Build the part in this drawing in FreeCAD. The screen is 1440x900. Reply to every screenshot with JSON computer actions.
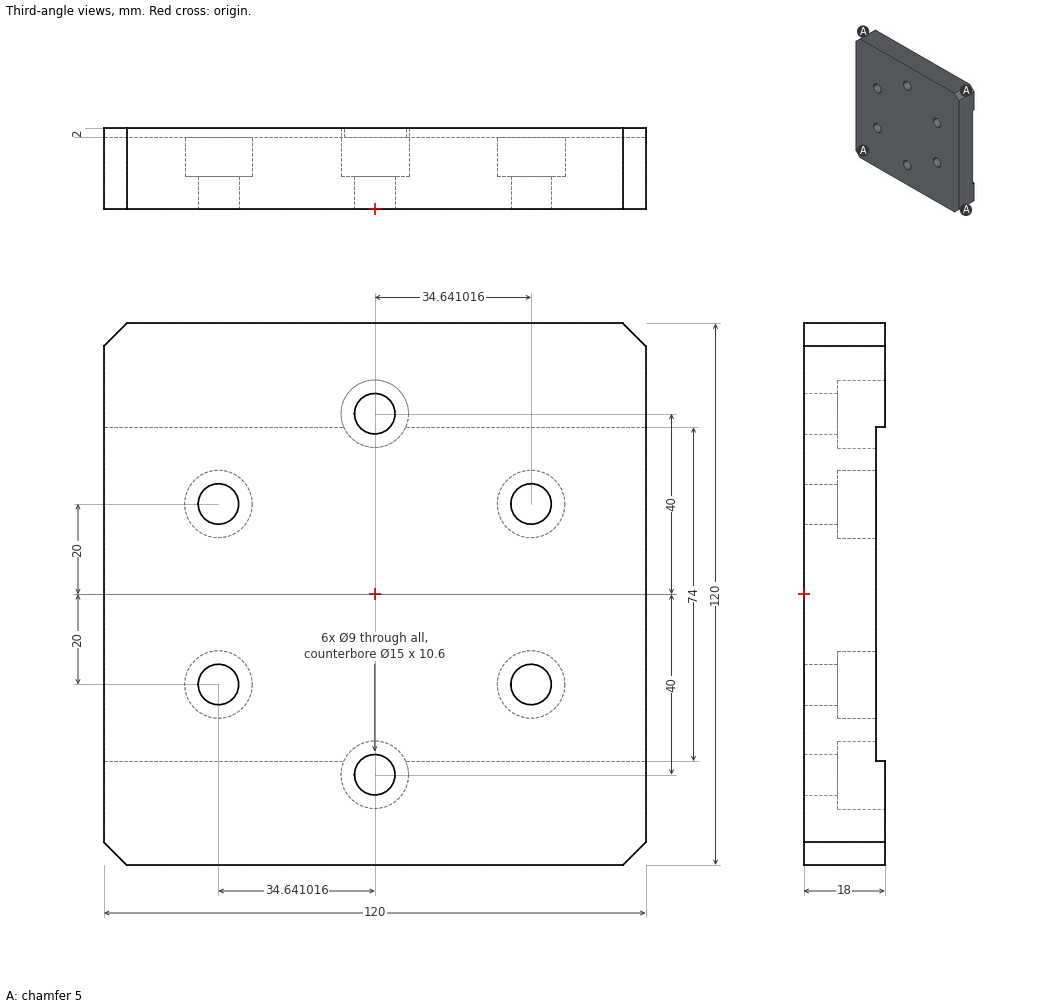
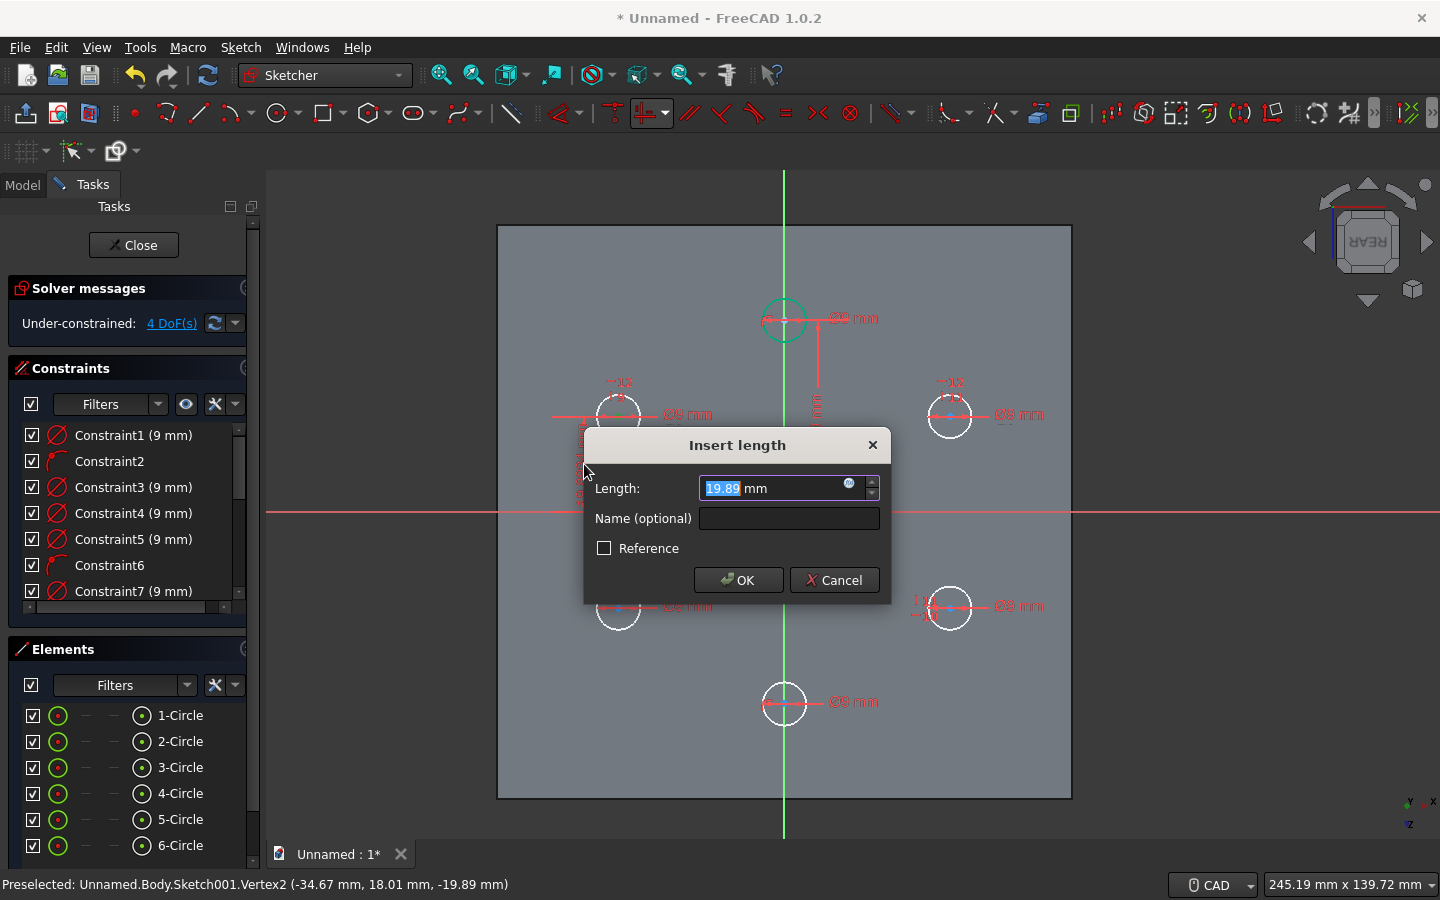
{"action": "type", "text": "20"}
{"action": "key", "text": "Return"}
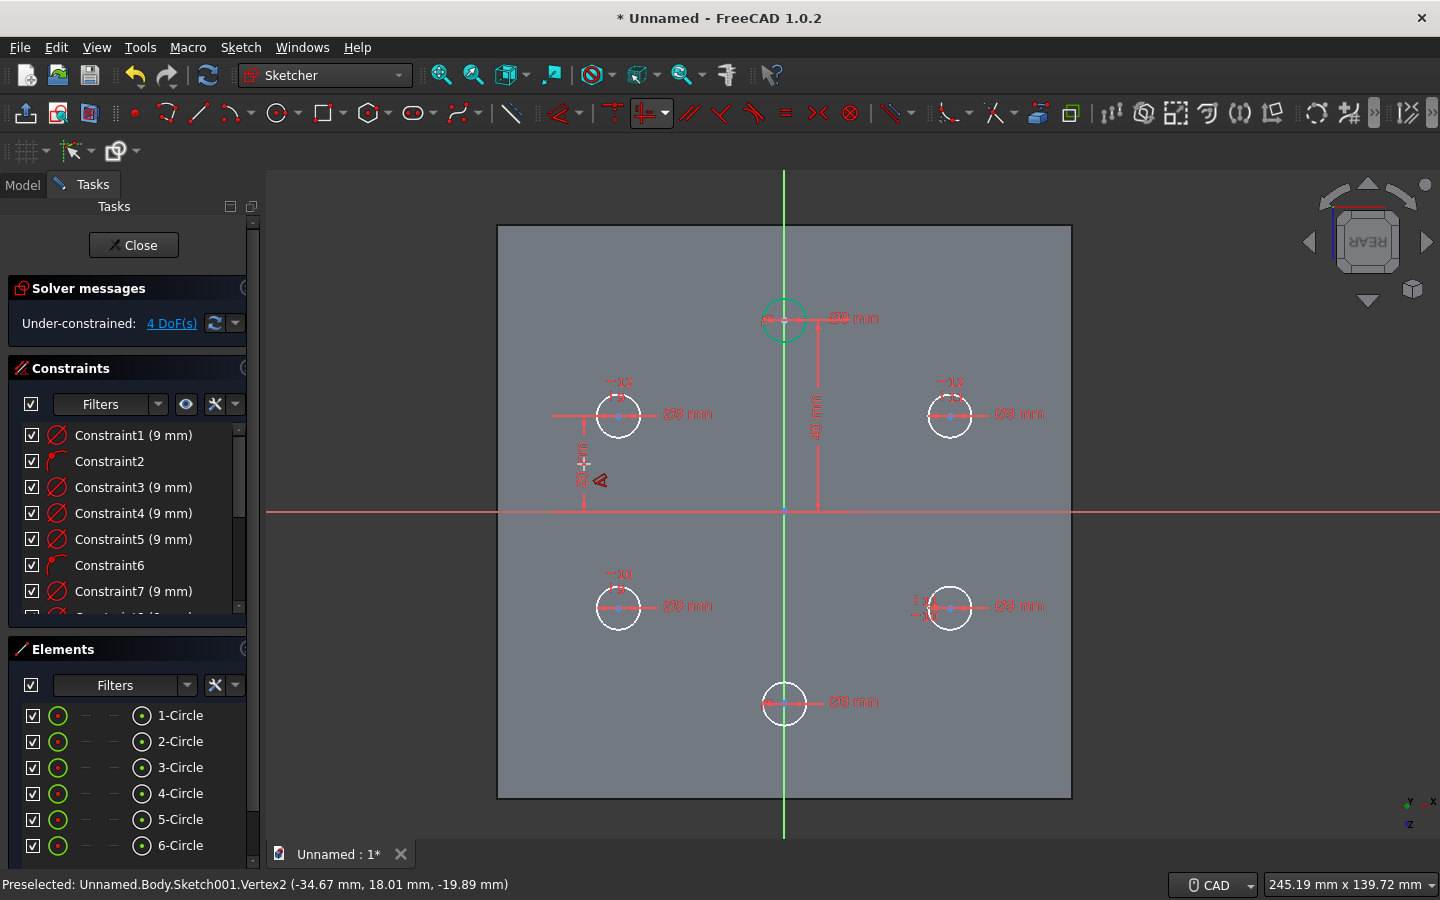
{"action": "left_click", "coordinate": [618, 608]}
{"action": "left_click", "coordinate": [584, 560]}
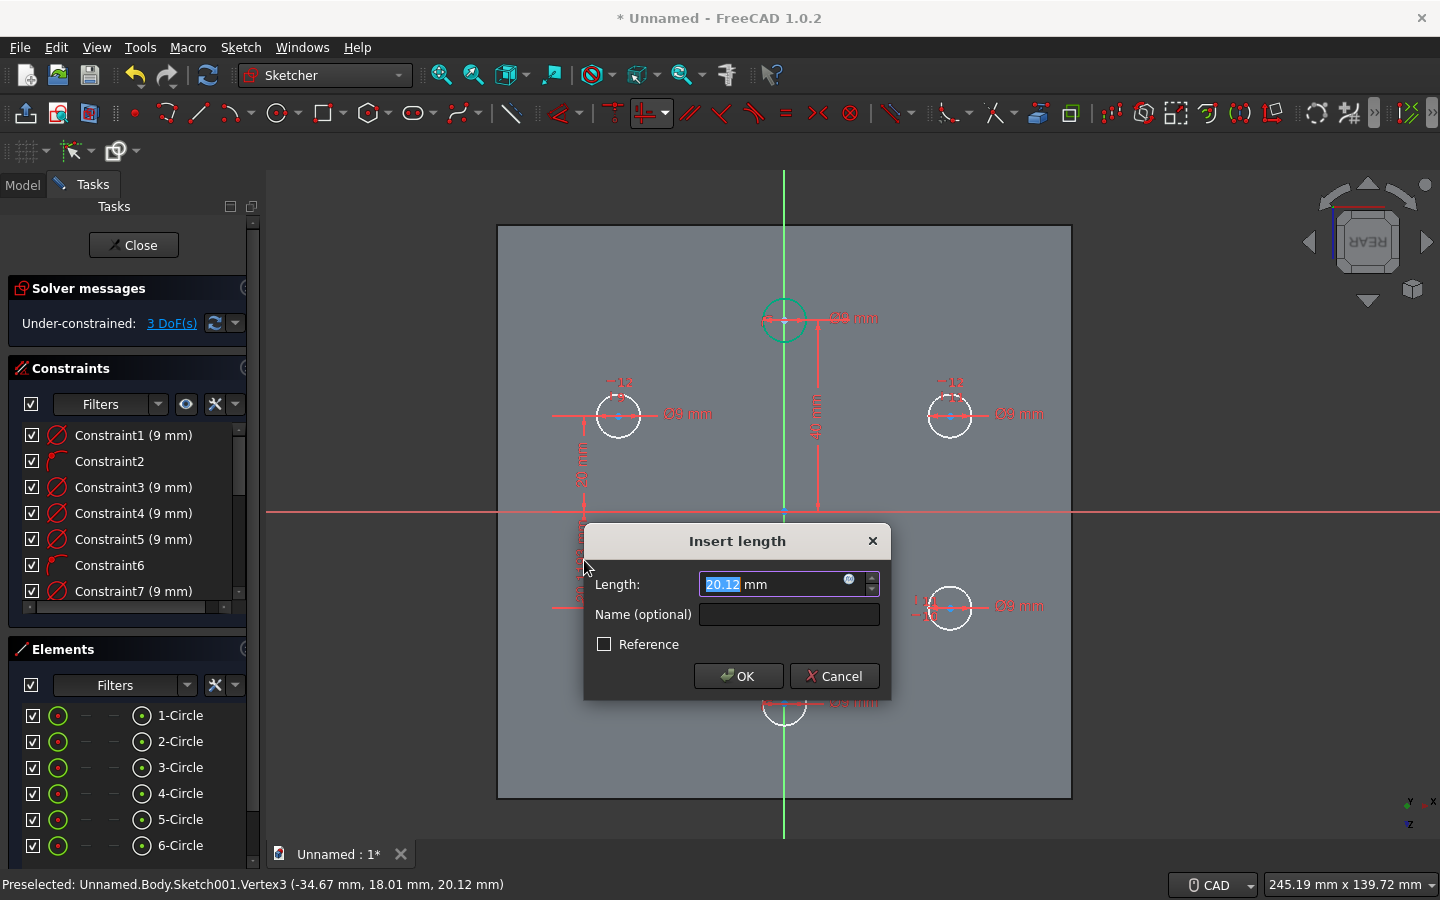
{"action": "type", "text": "20"}
{"action": "key", "text": "Return"}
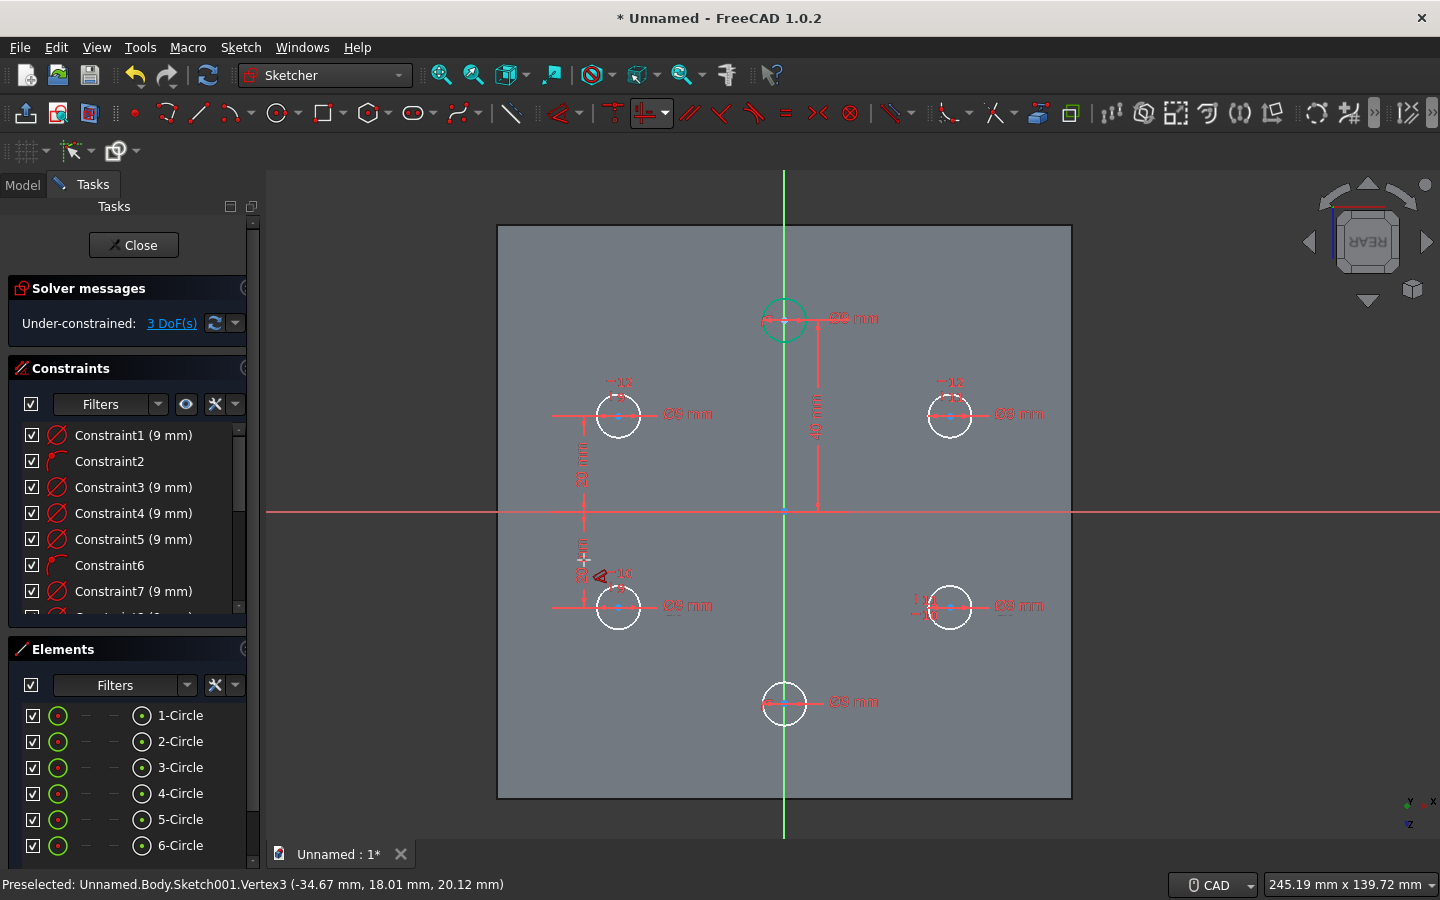
{"action": "left_click", "coordinate": [784, 704]}
{"action": "left_click", "coordinate": [818, 608]}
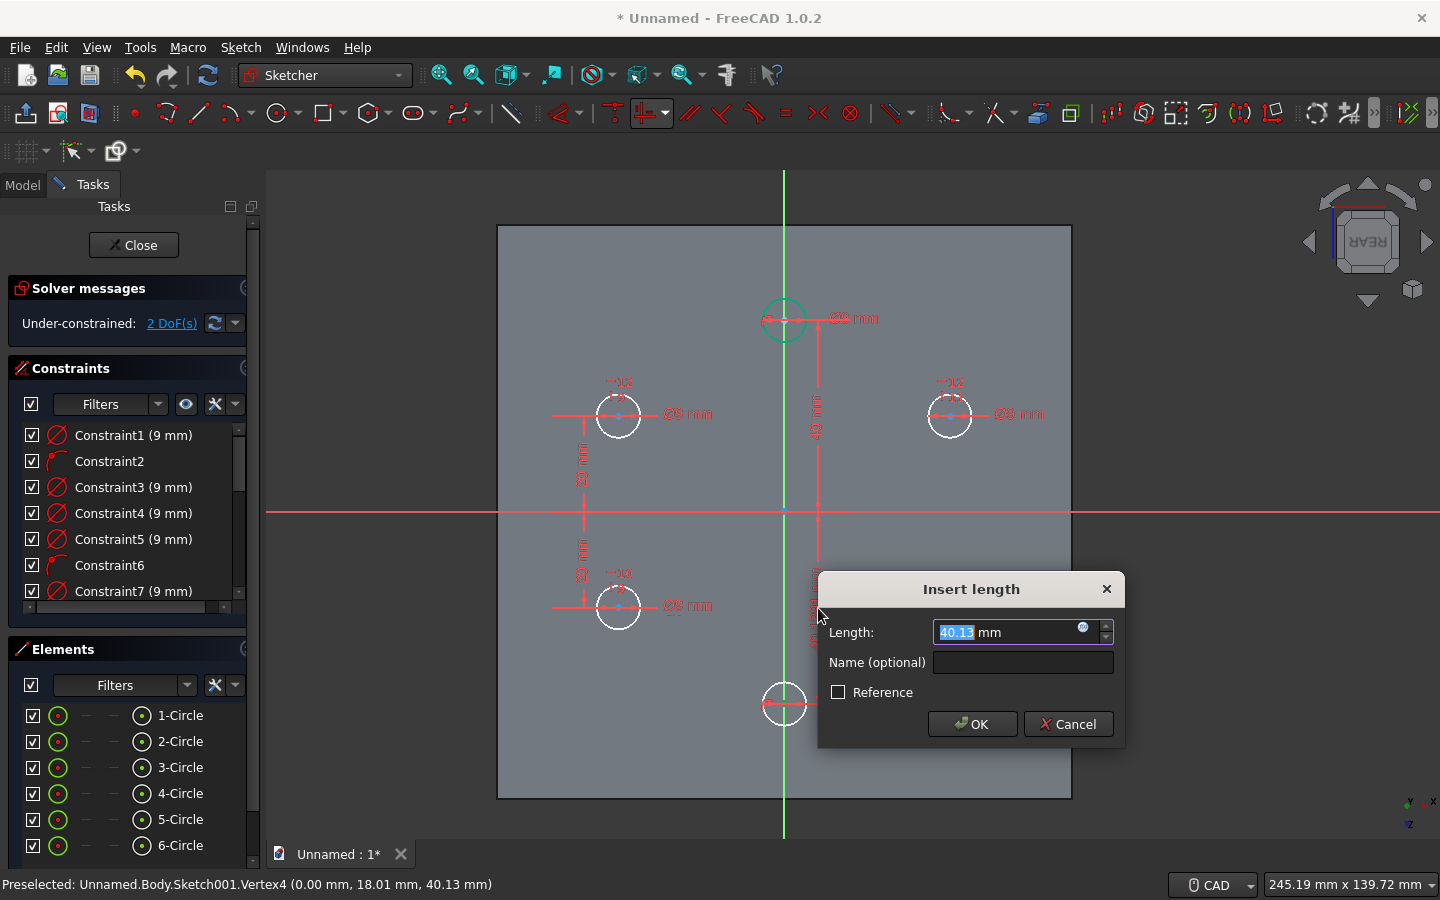
{"action": "type", "text": "40"}
{"action": "key", "text": "Return"}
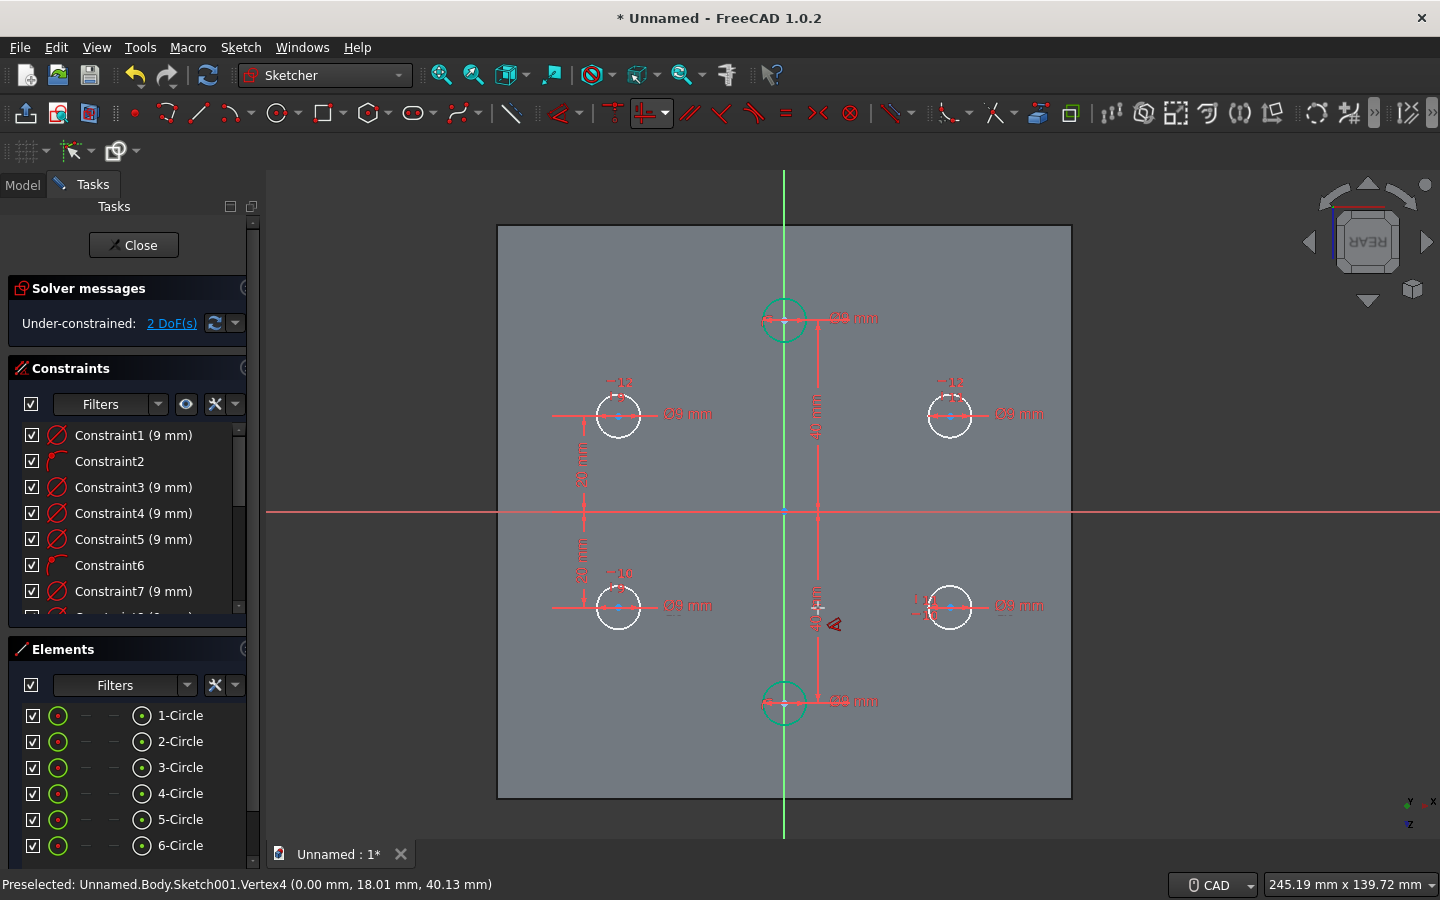
{"action": "left_click", "coordinate": [618, 416]}
{"action": "left_click", "coordinate": [701, 382]}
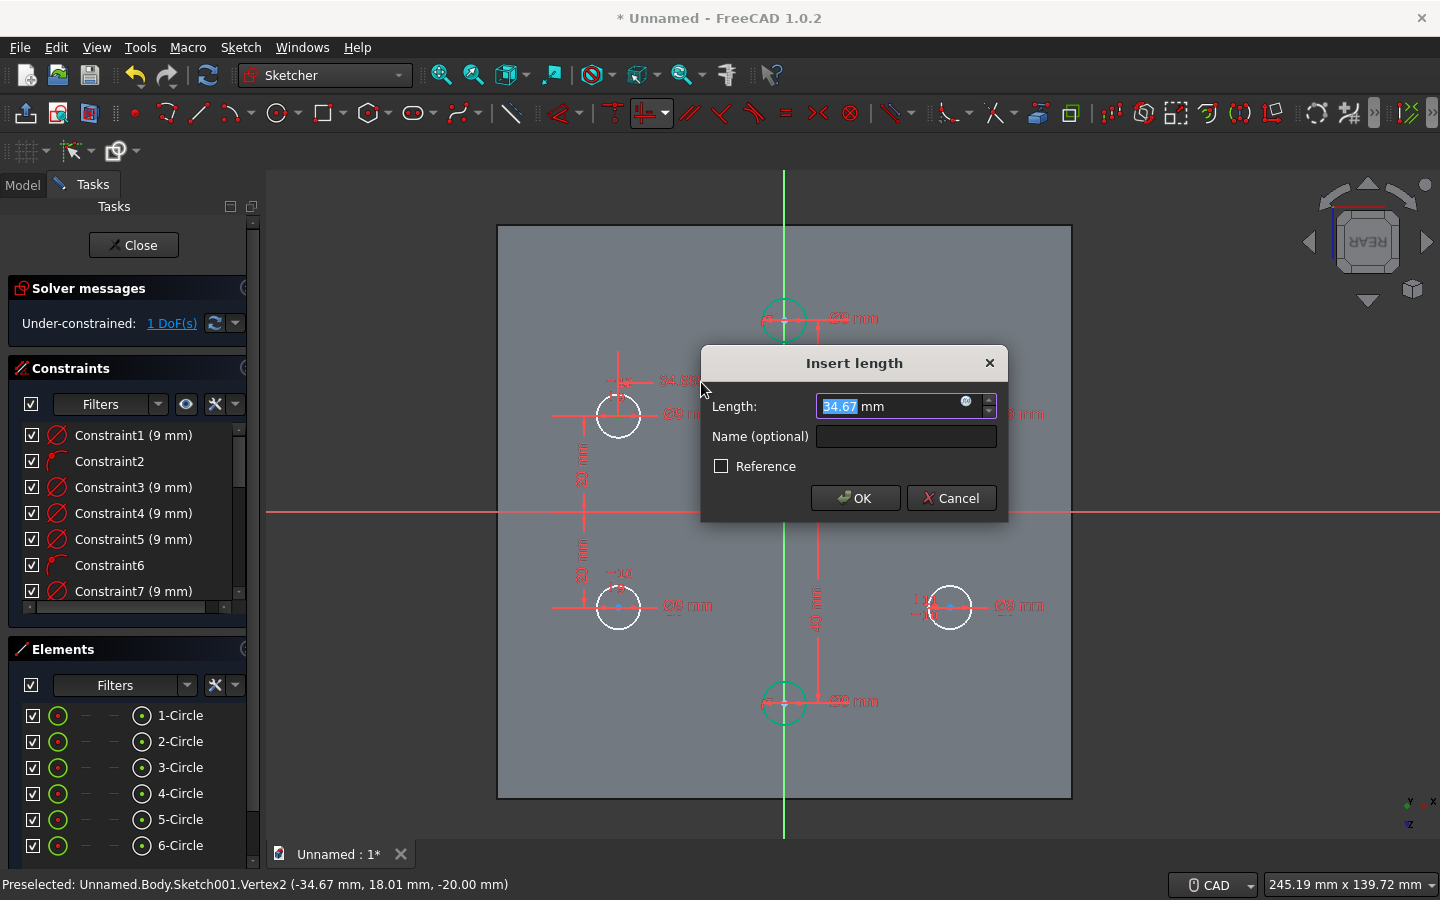
{"action": "type", "text": "34.641016"}
{"action": "key", "text": "Return"}